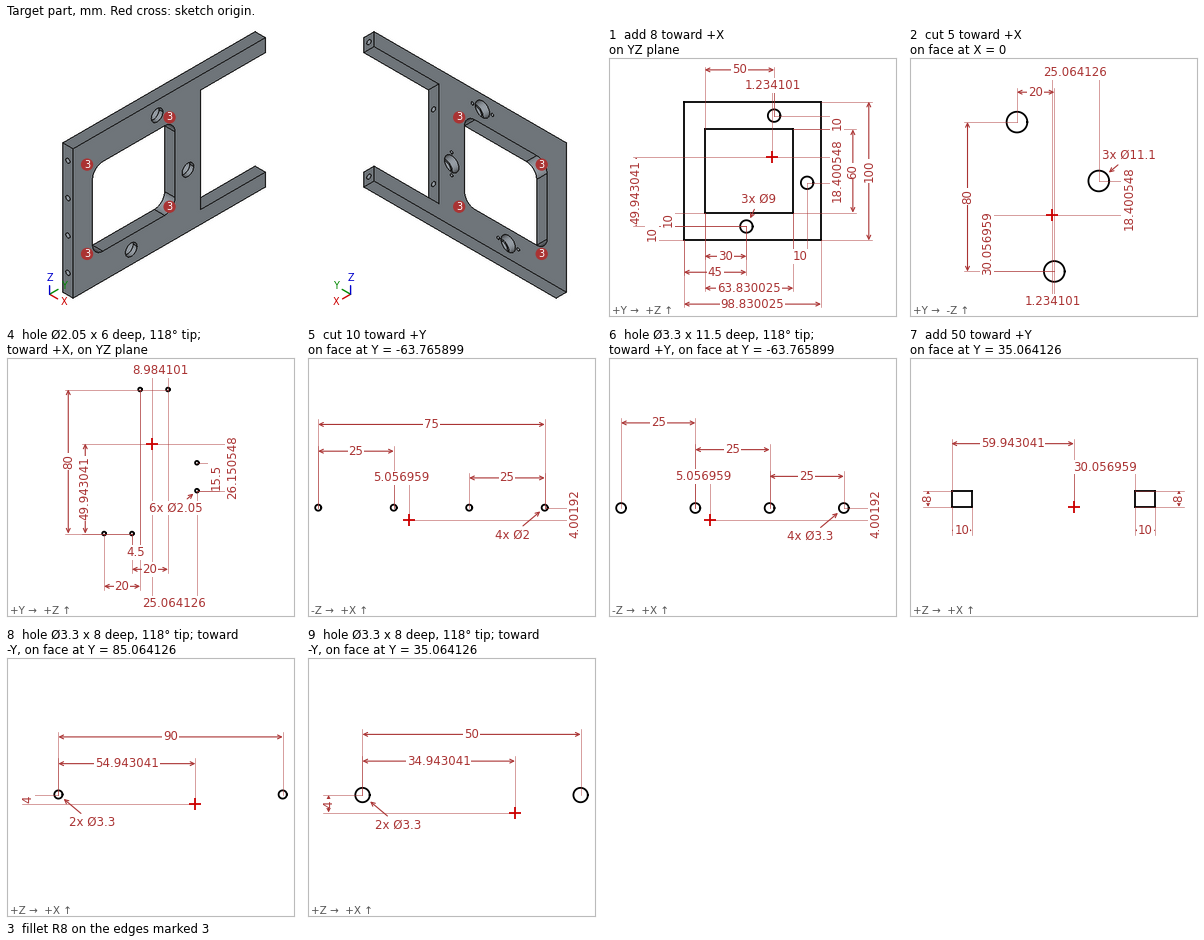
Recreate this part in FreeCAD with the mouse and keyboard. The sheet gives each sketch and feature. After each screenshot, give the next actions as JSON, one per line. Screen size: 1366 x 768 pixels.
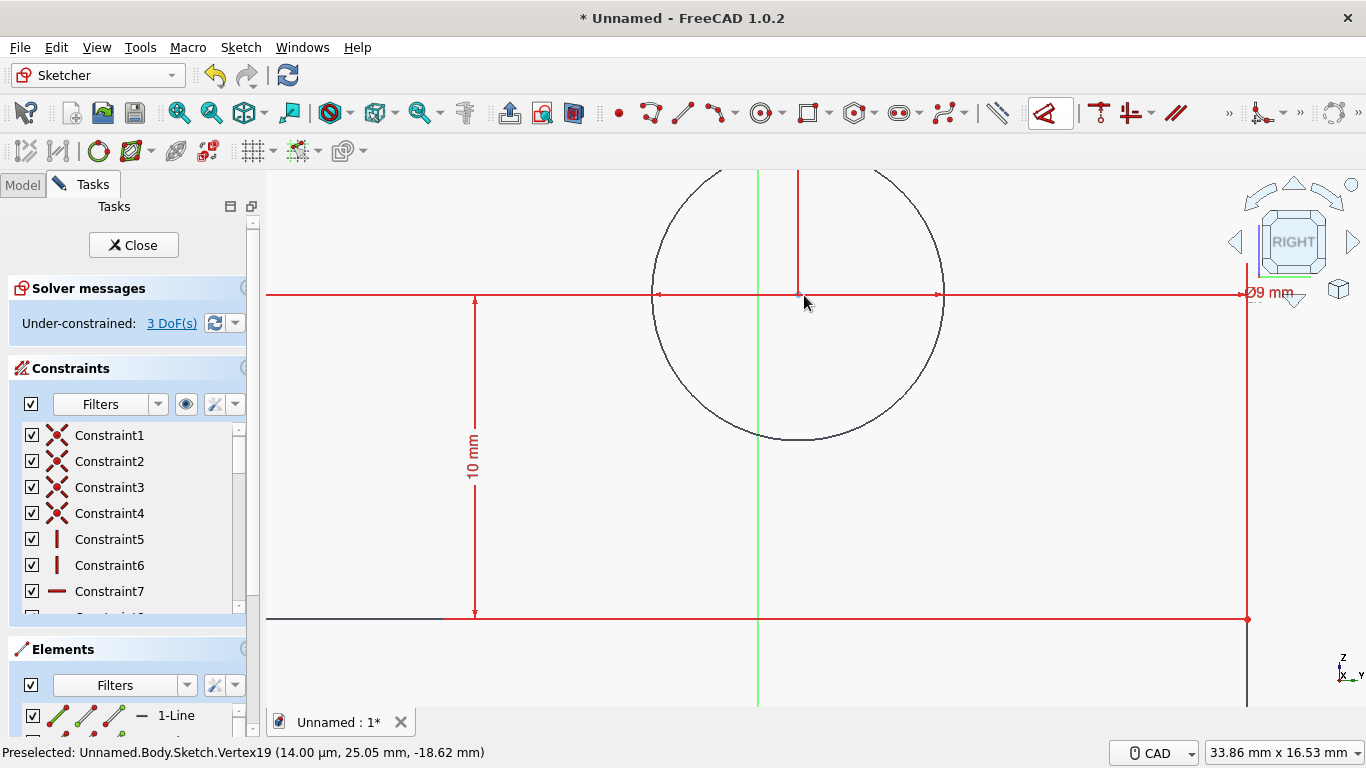
{"action": "left_click", "coordinate": [798, 295]}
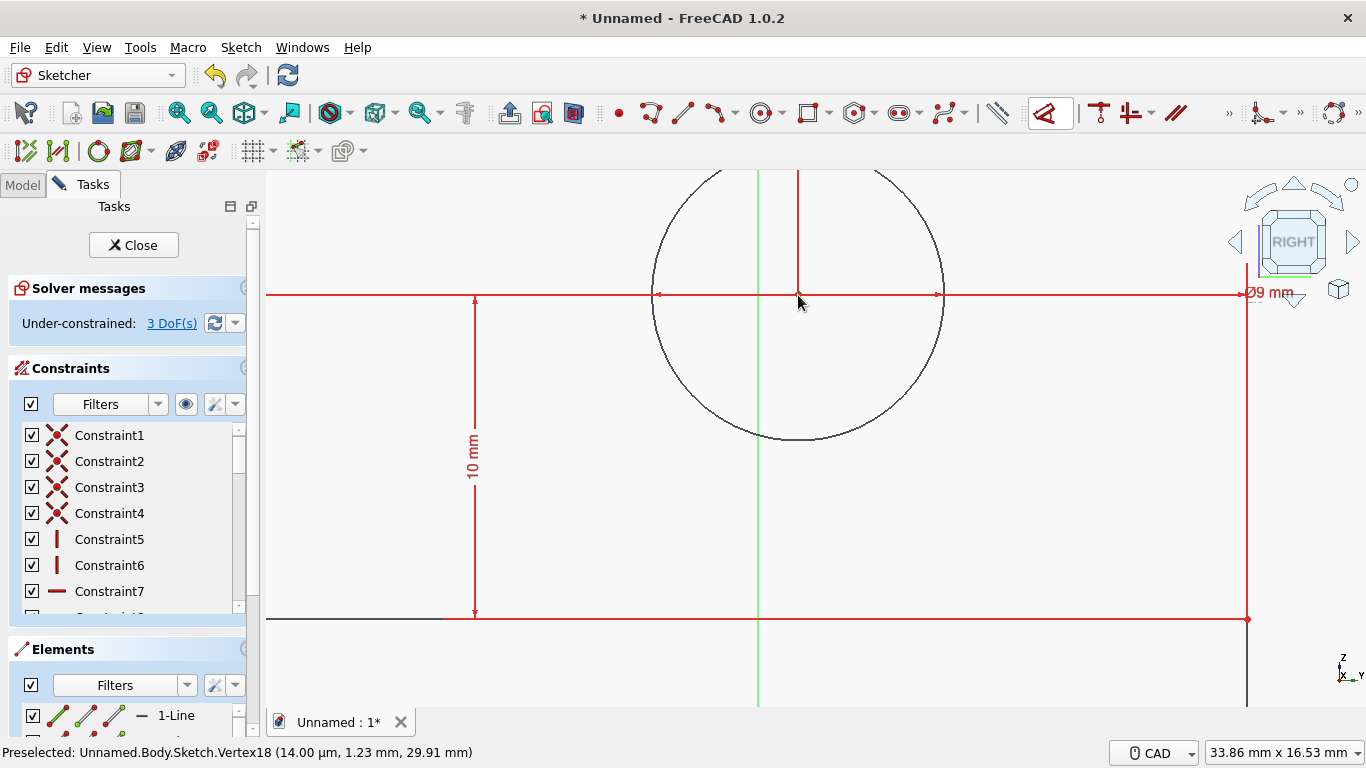
{"action": "key", "text": "l"}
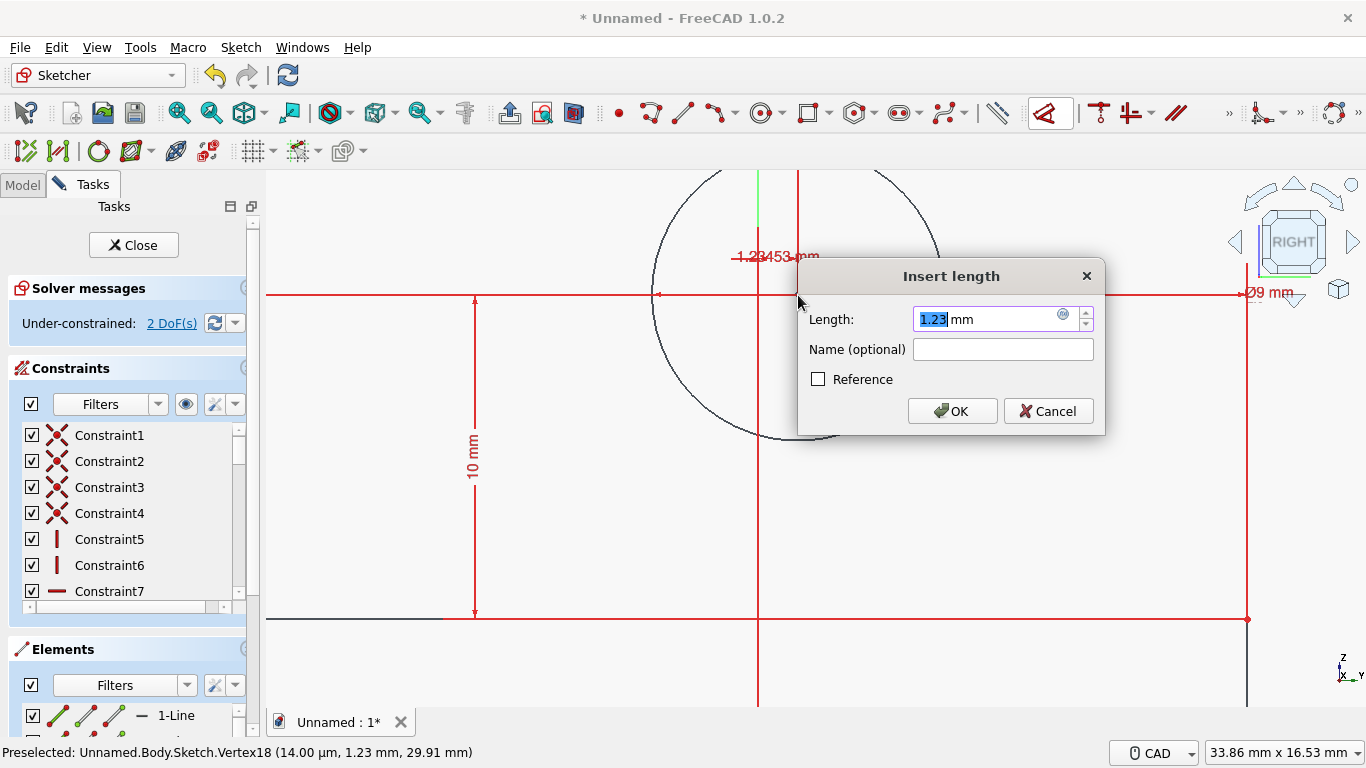
{"action": "type", "text": "1.234101"}
{"action": "key", "text": "Return"}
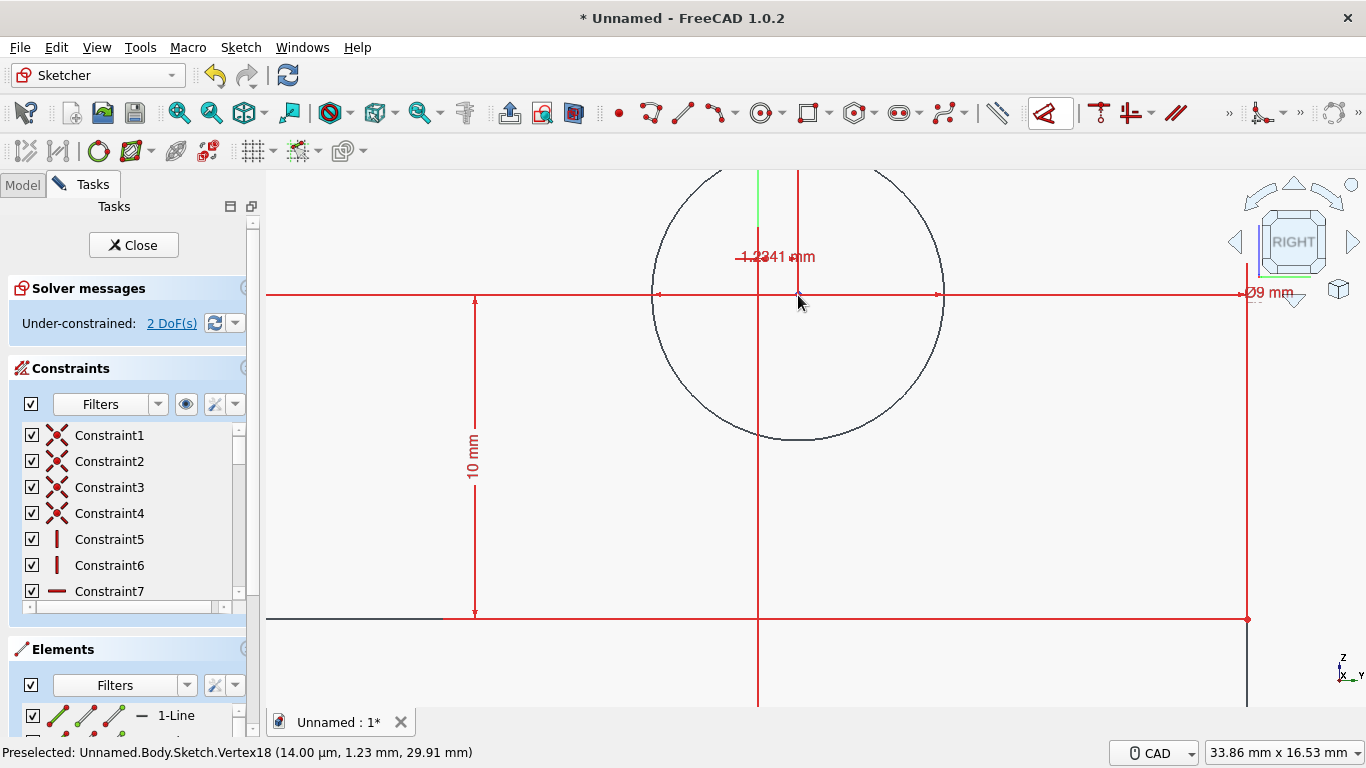
{"action": "scroll", "coordinate": [804, 295], "scroll_direction": "down", "scroll_amount": 11}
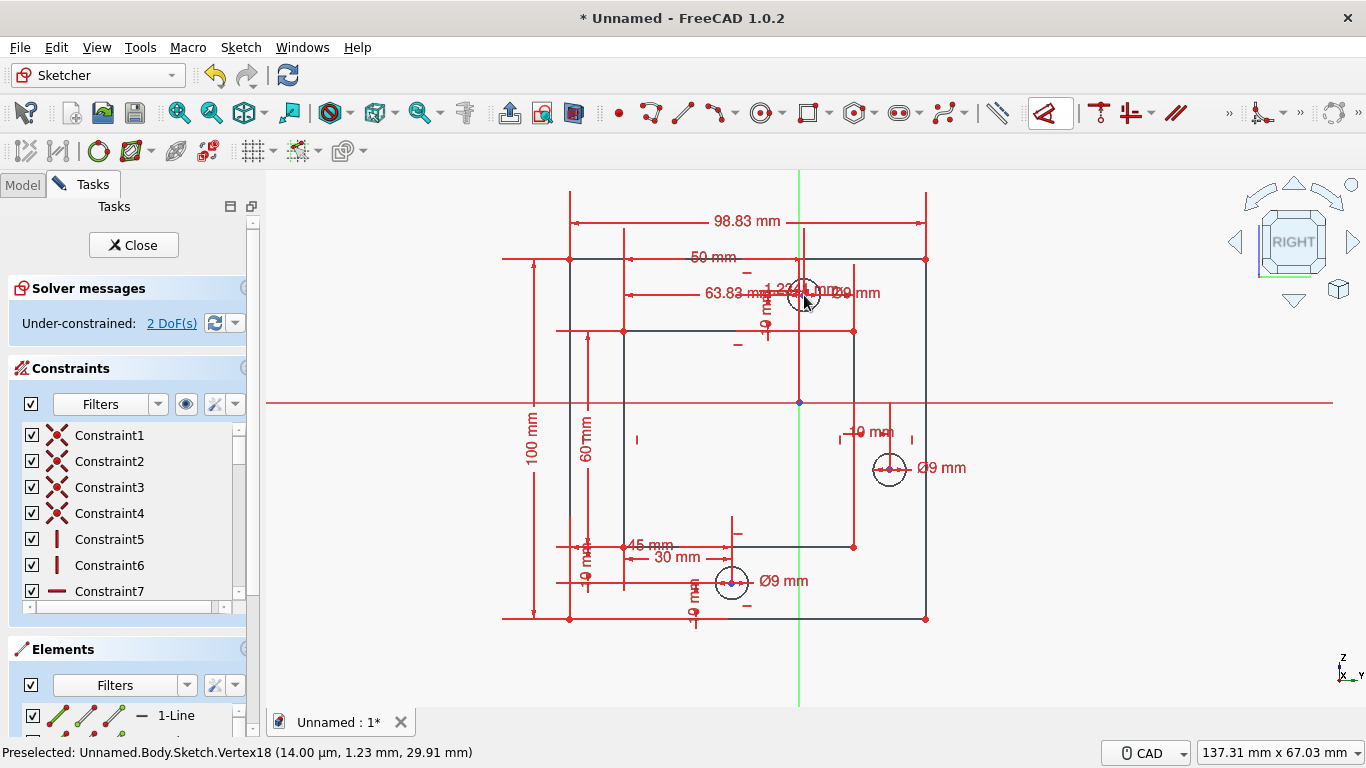
{"action": "left_click", "coordinate": [732, 583]}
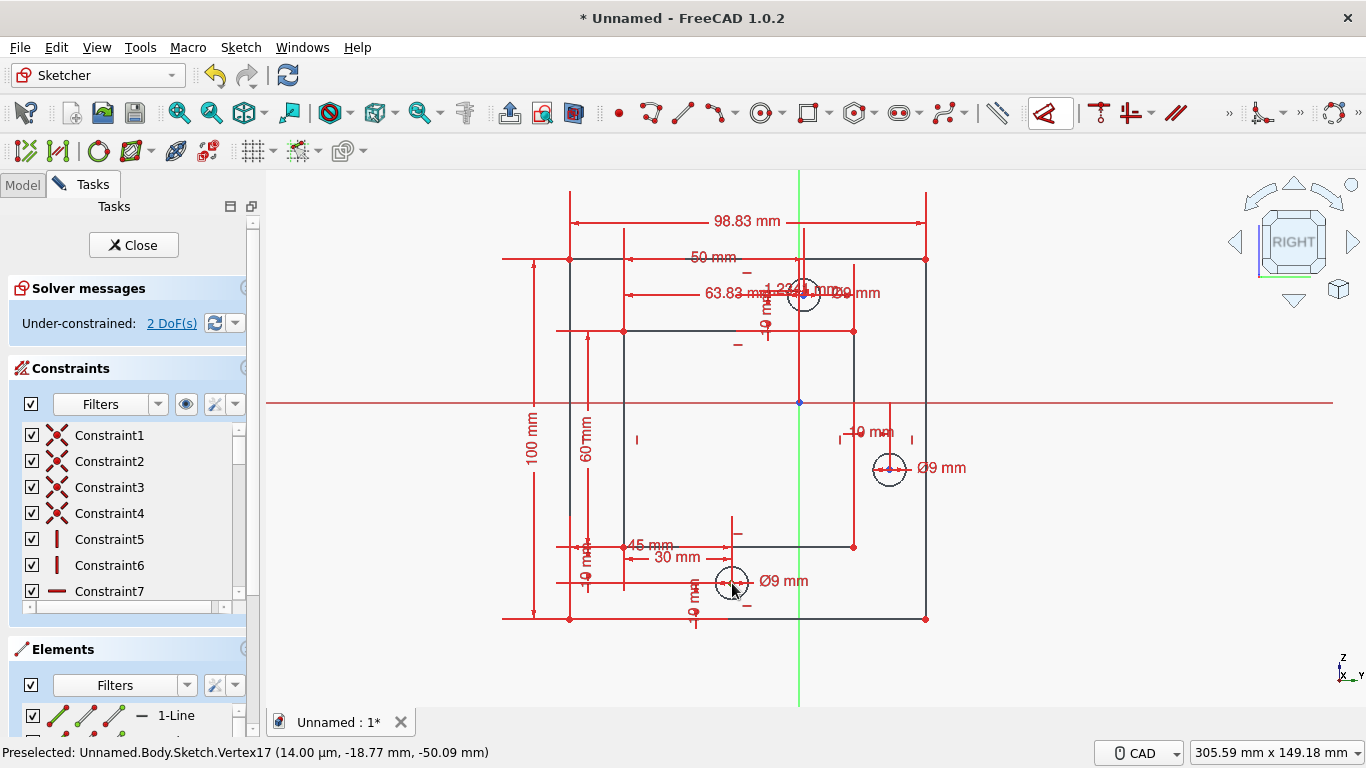
{"action": "key", "text": "i"}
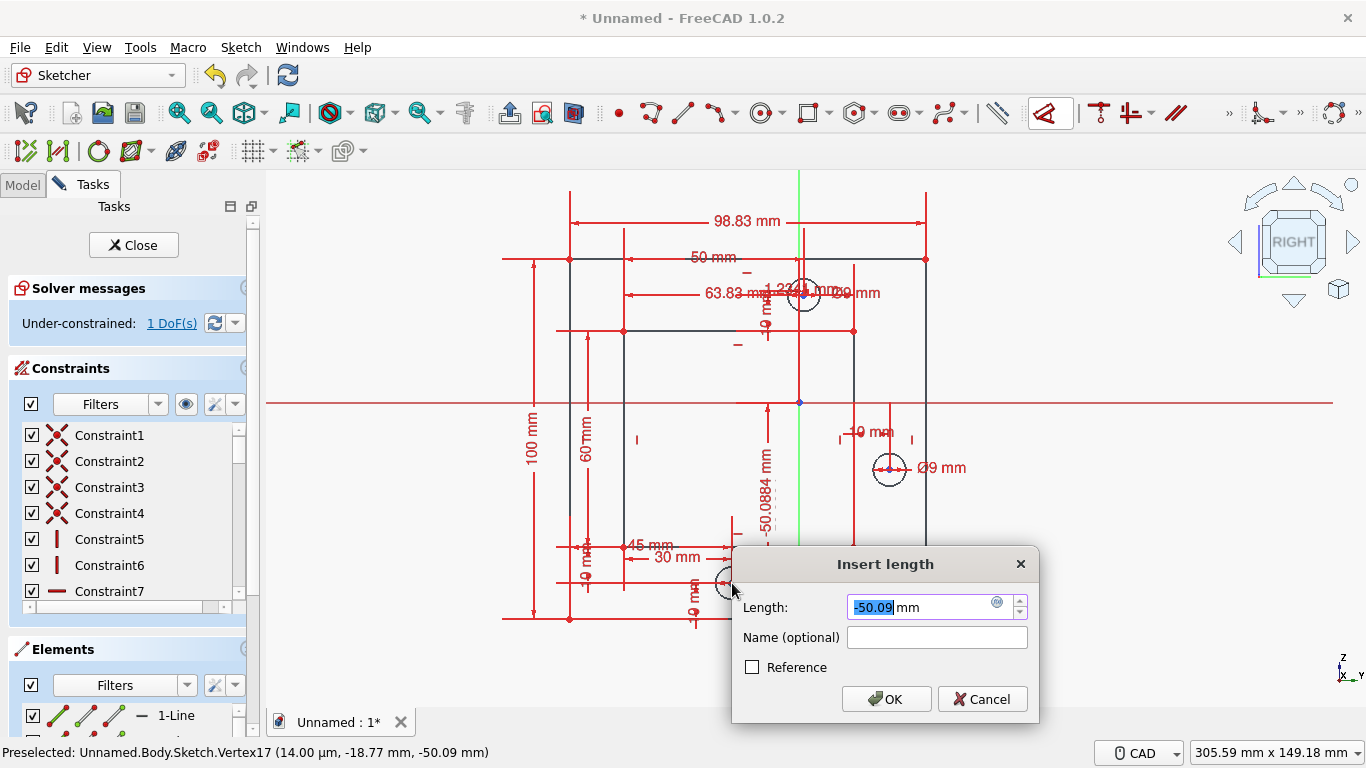
{"action": "type", "text": "-49.943041"}
{"action": "key", "text": "Return"}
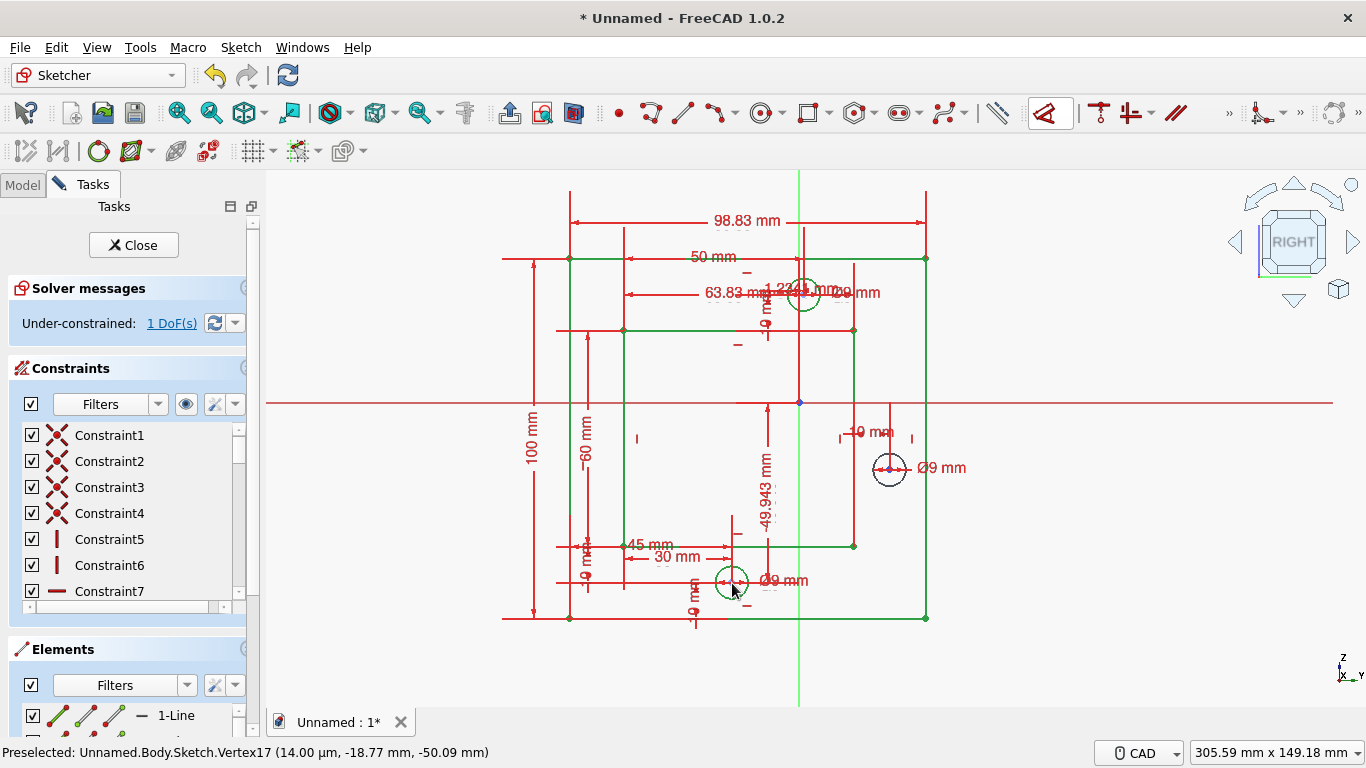
{"action": "left_click", "coordinate": [890, 470]}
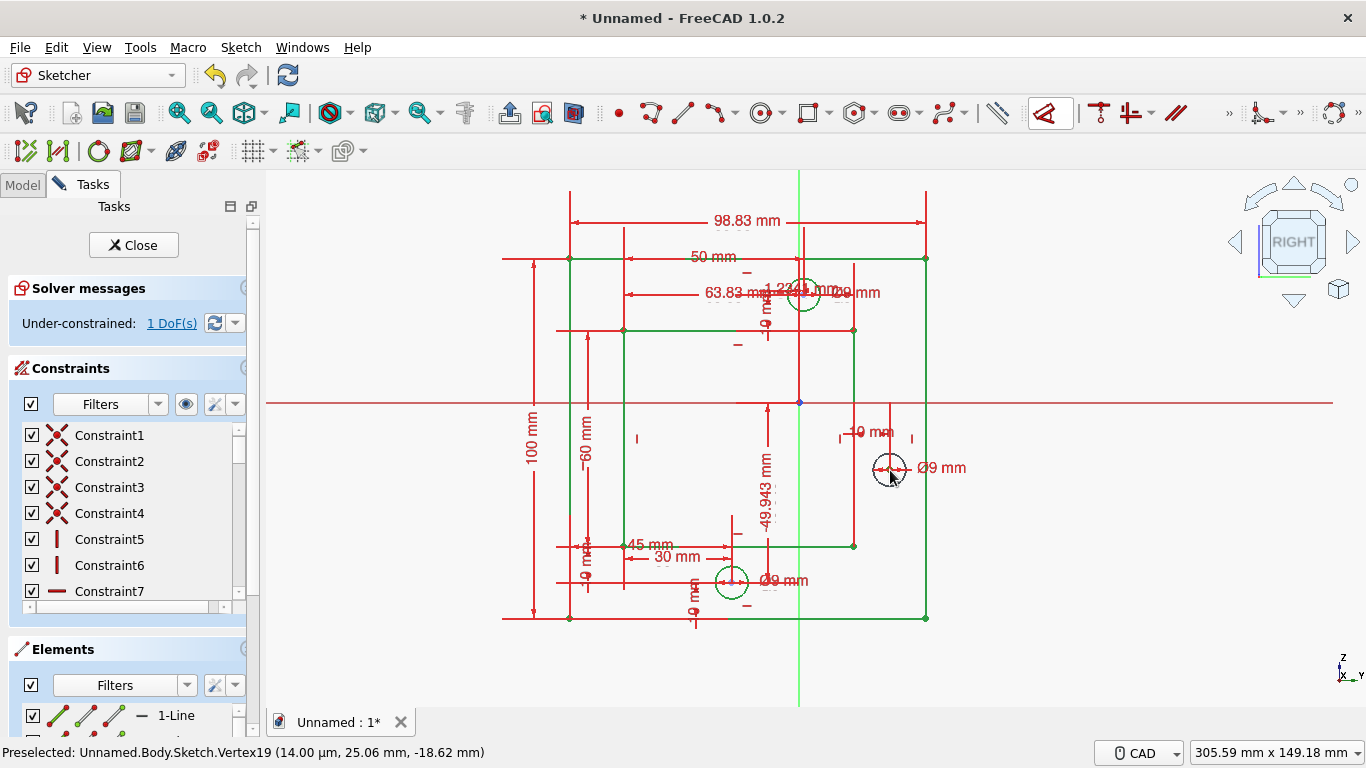
{"action": "left_click", "coordinate": [1068, 114]}